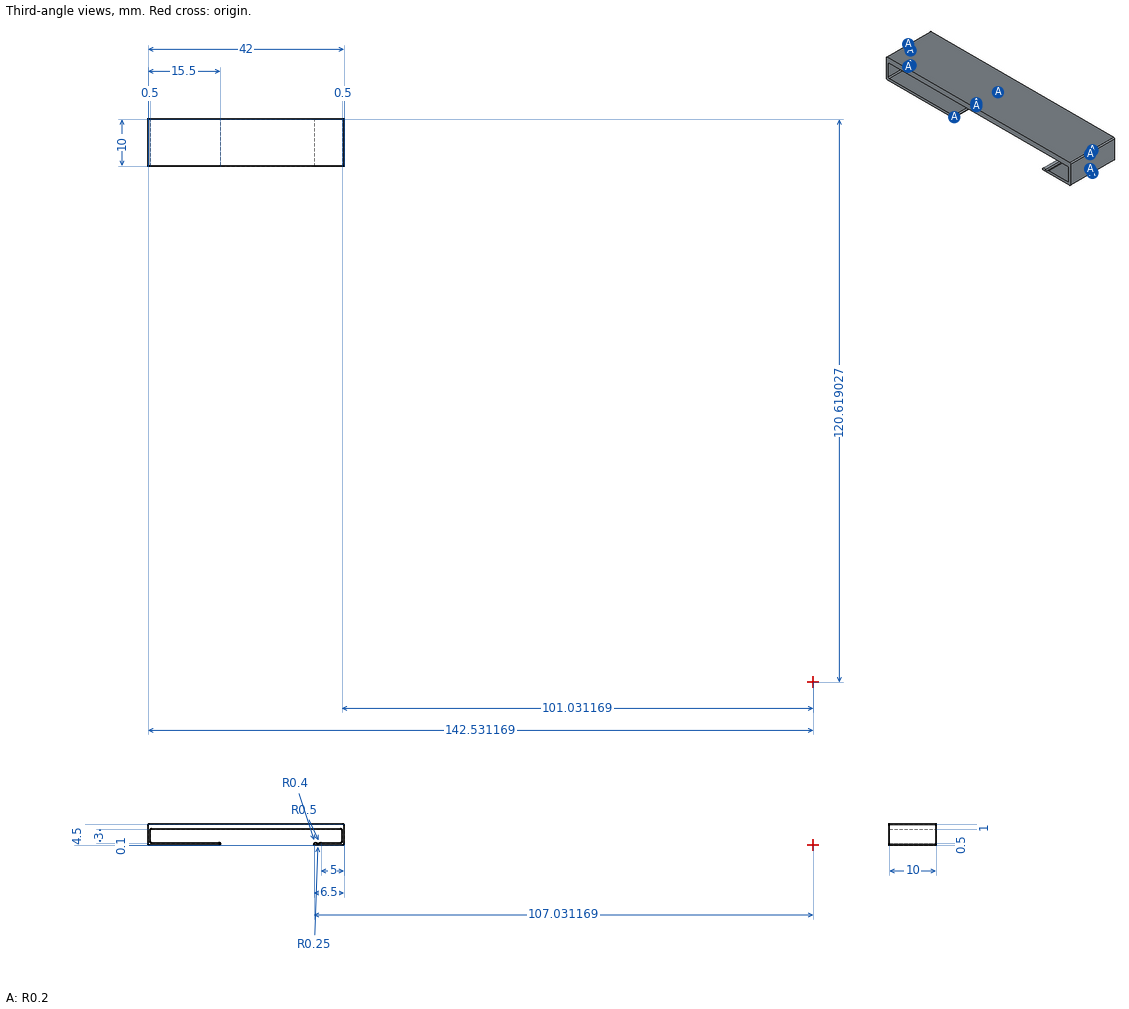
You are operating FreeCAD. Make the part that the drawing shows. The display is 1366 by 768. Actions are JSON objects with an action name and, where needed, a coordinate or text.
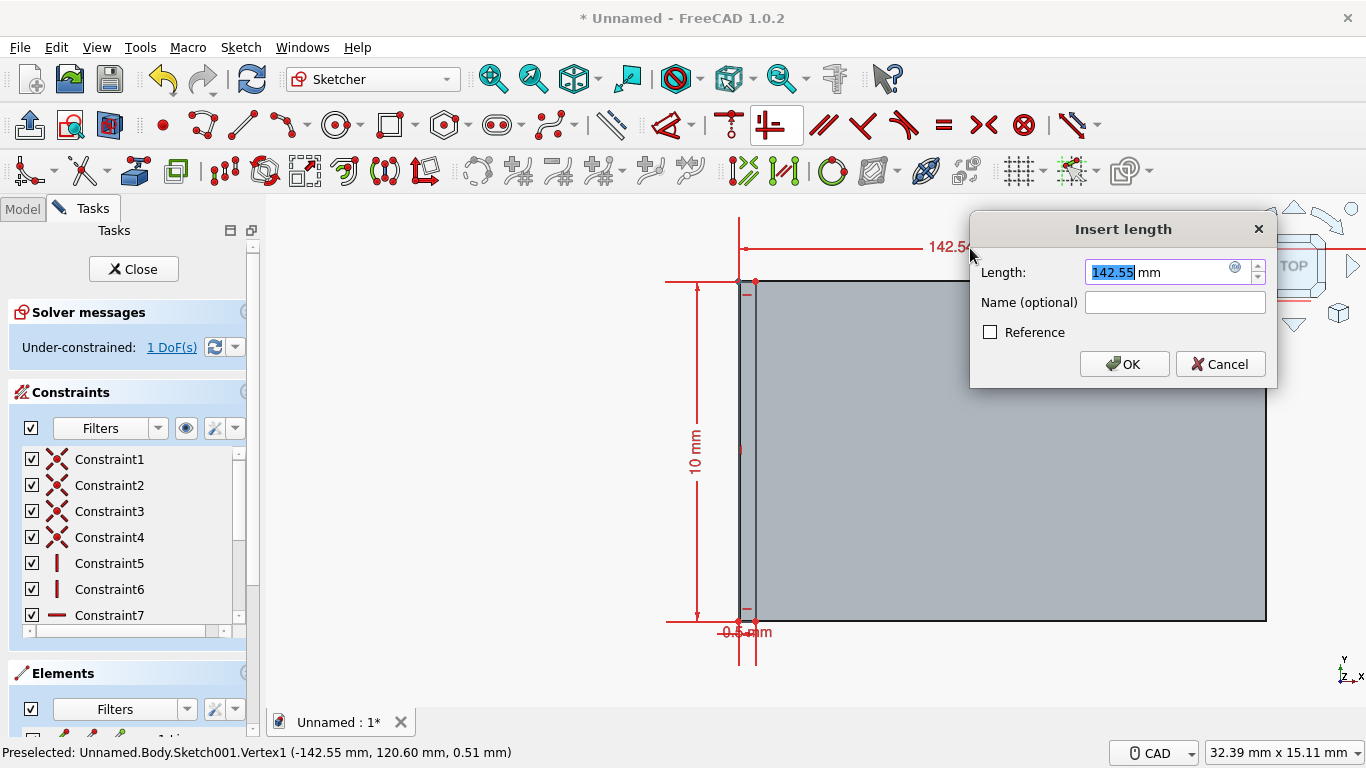
{"action": "type", "text": "142.531169"}
{"action": "key", "text": "Return"}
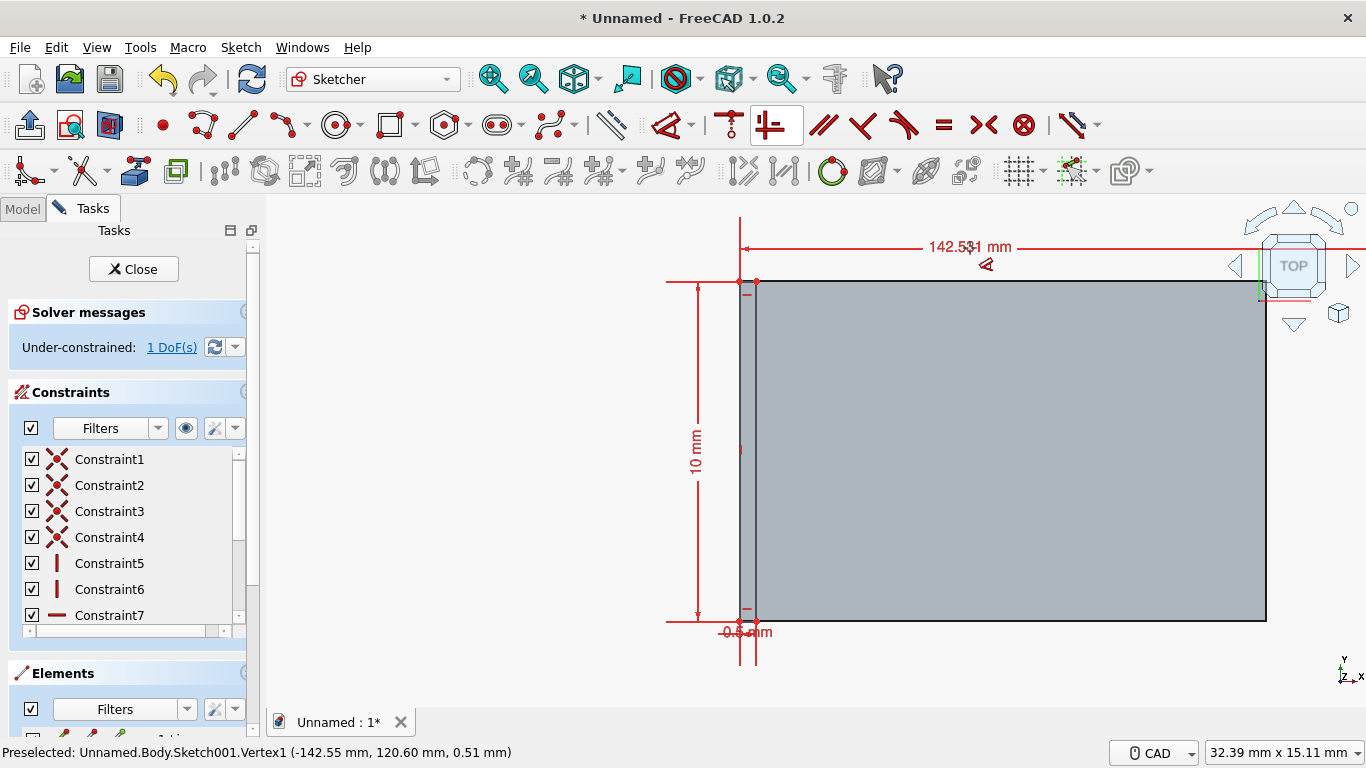
{"action": "left_click", "coordinate": [740, 282]}
{"action": "left_click", "coordinate": [706, 480]}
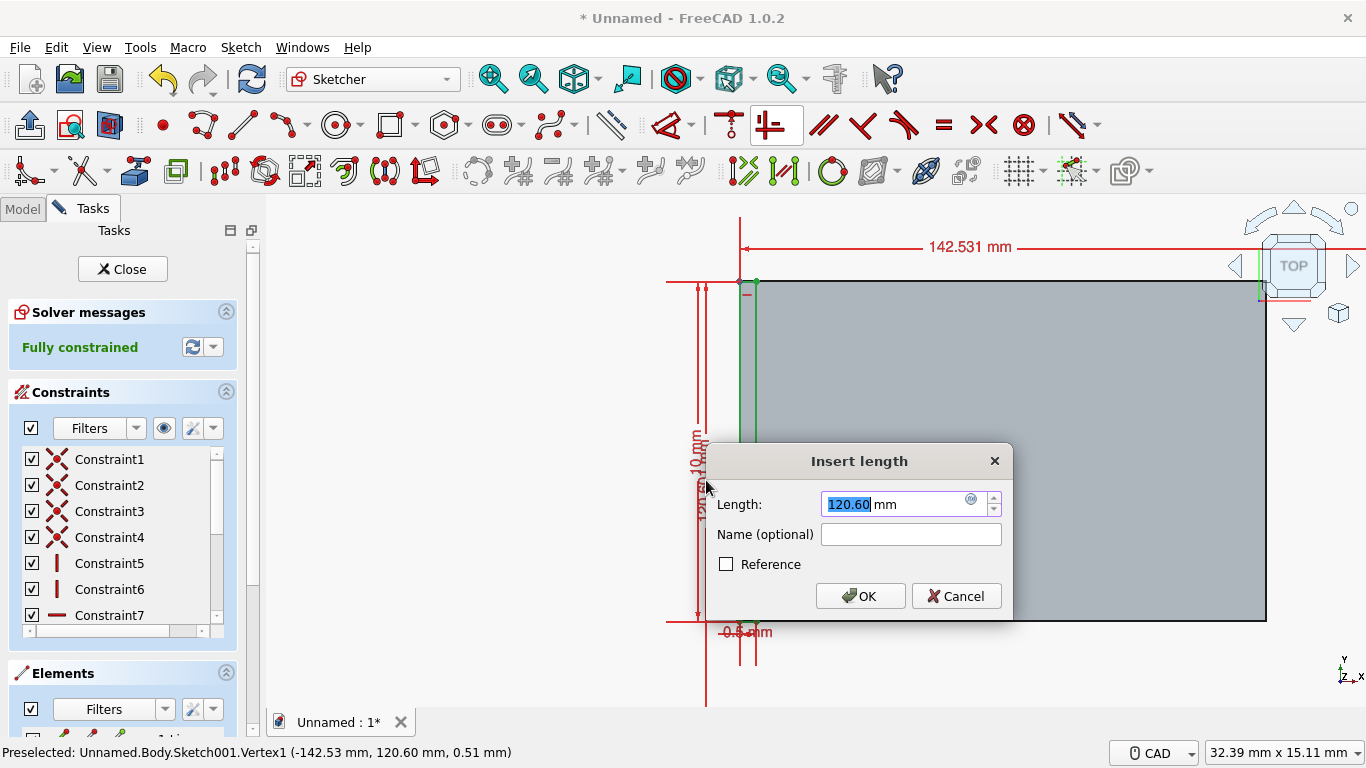
{"action": "type", "text": "120.619027"}
{"action": "key", "text": "Return"}
{"action": "key", "text": "Escape"}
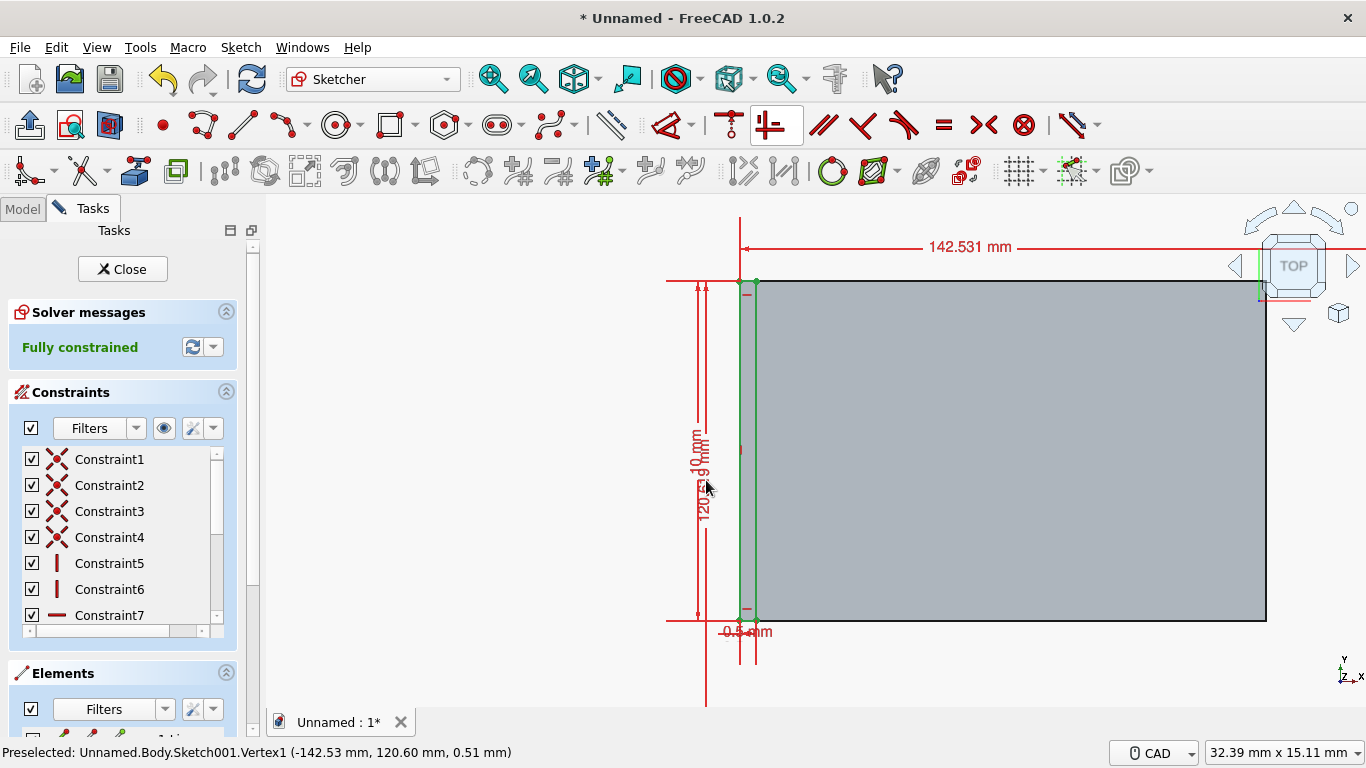
{"action": "left_click", "coordinate": [123, 269]}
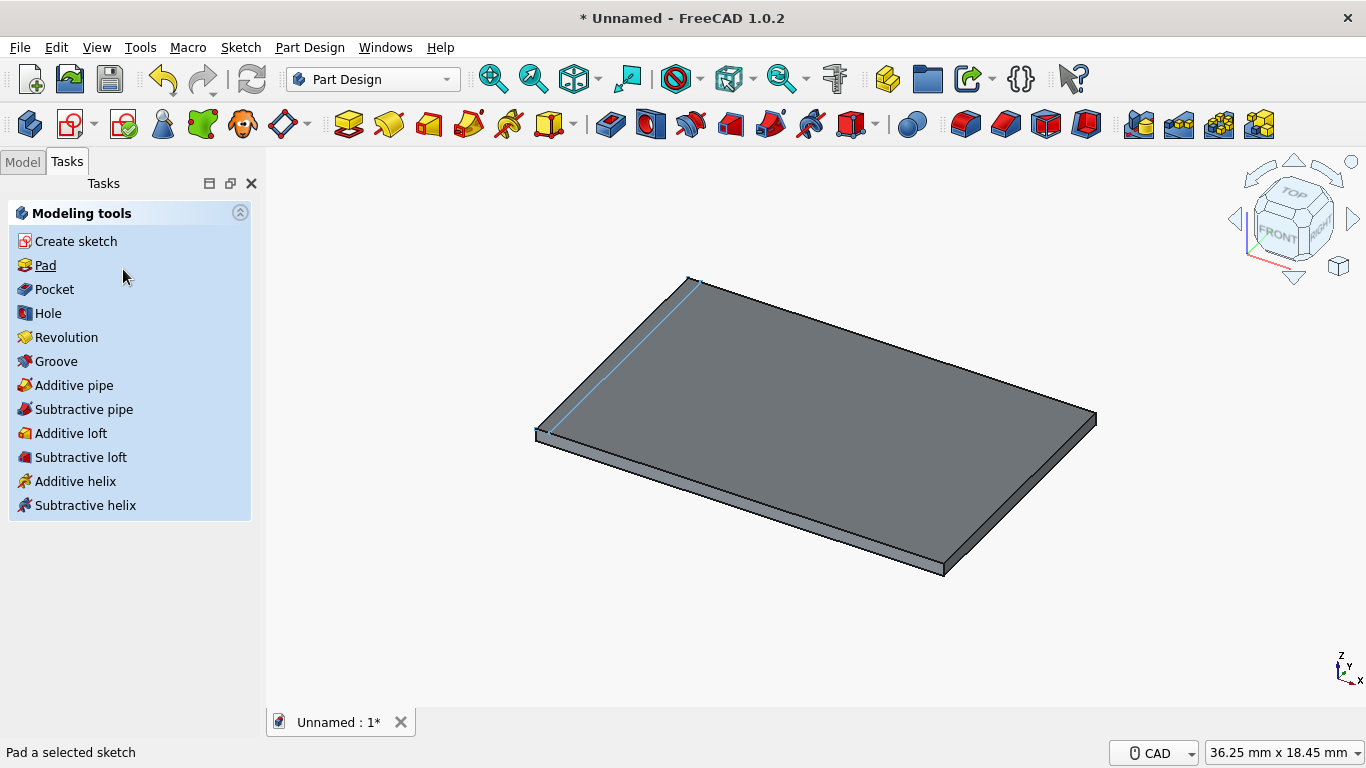
{"action": "left_click", "coordinate": [350, 124]}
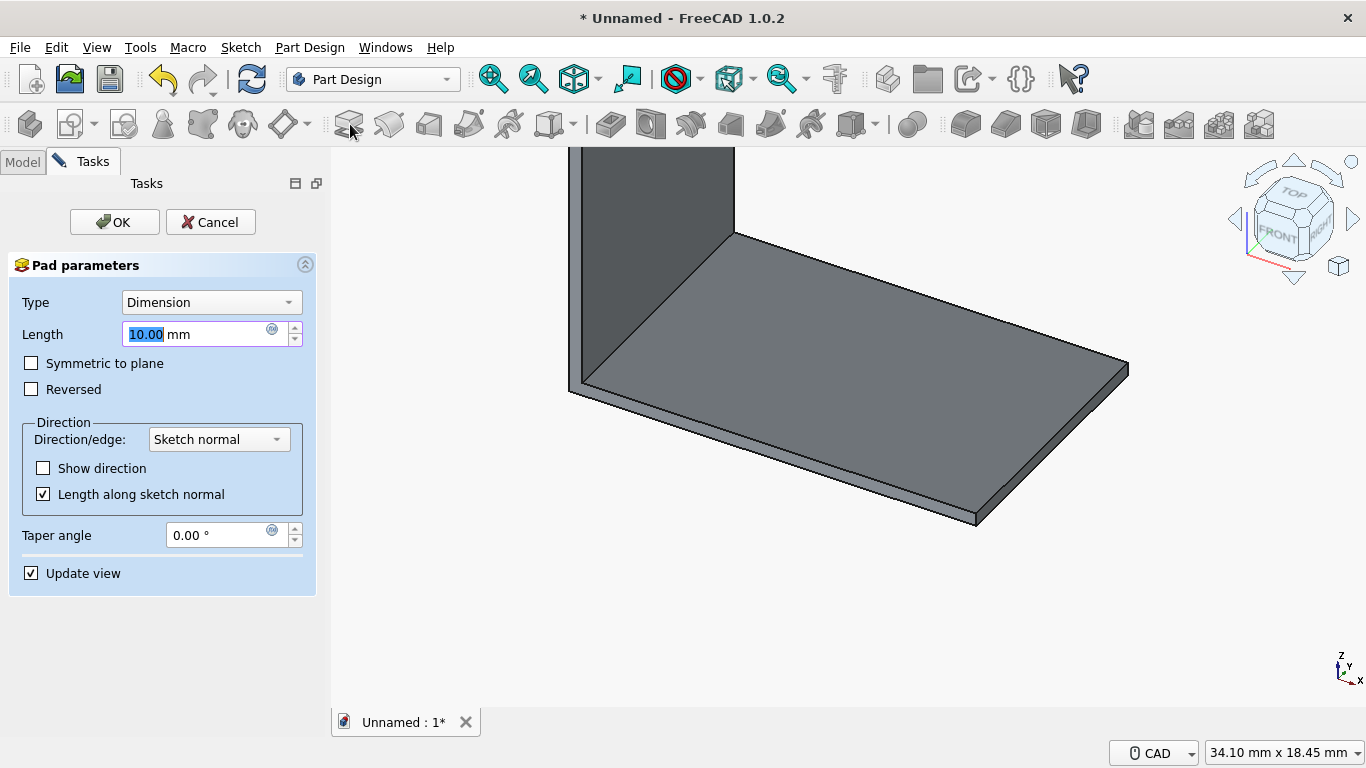
{"action": "type", "text": "3"}
{"action": "key", "text": "Tab"}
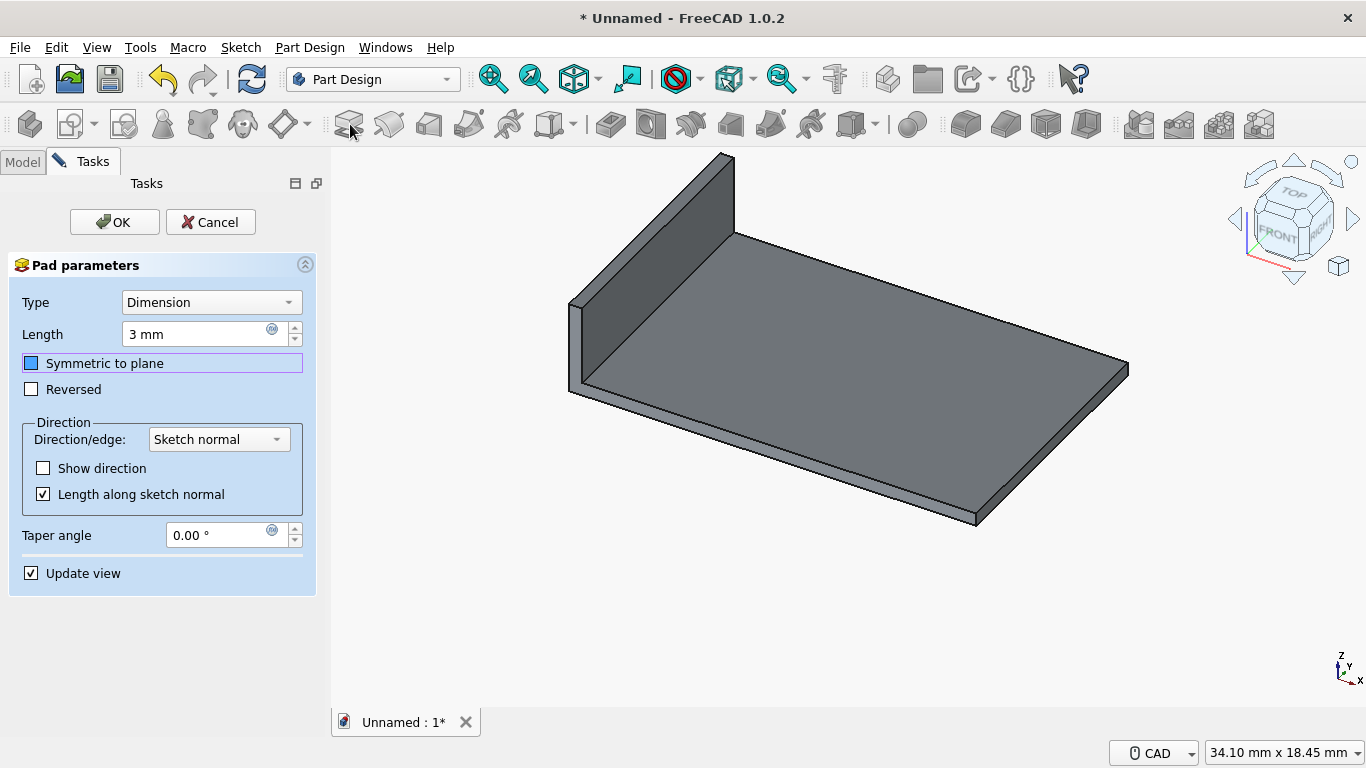
{"action": "left_click", "coordinate": [115, 222]}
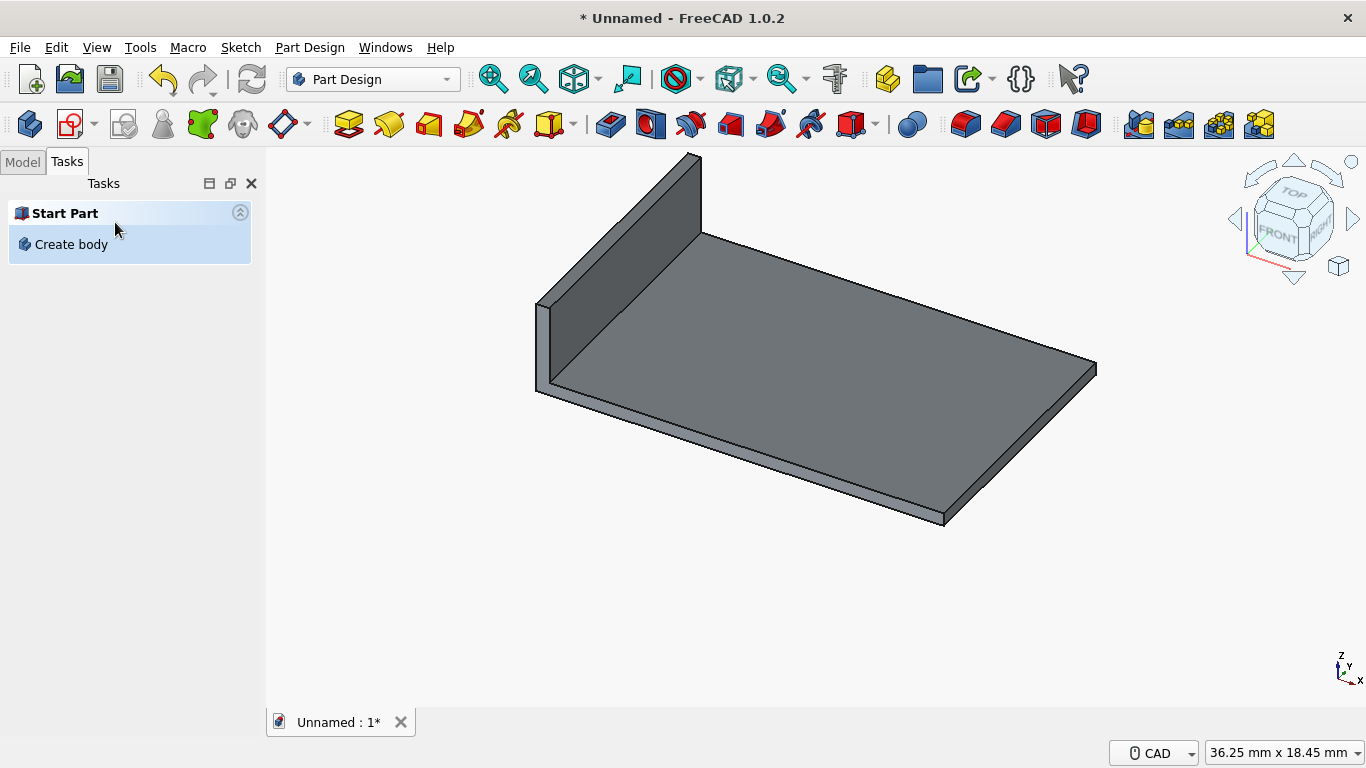
{"action": "key", "text": "0"}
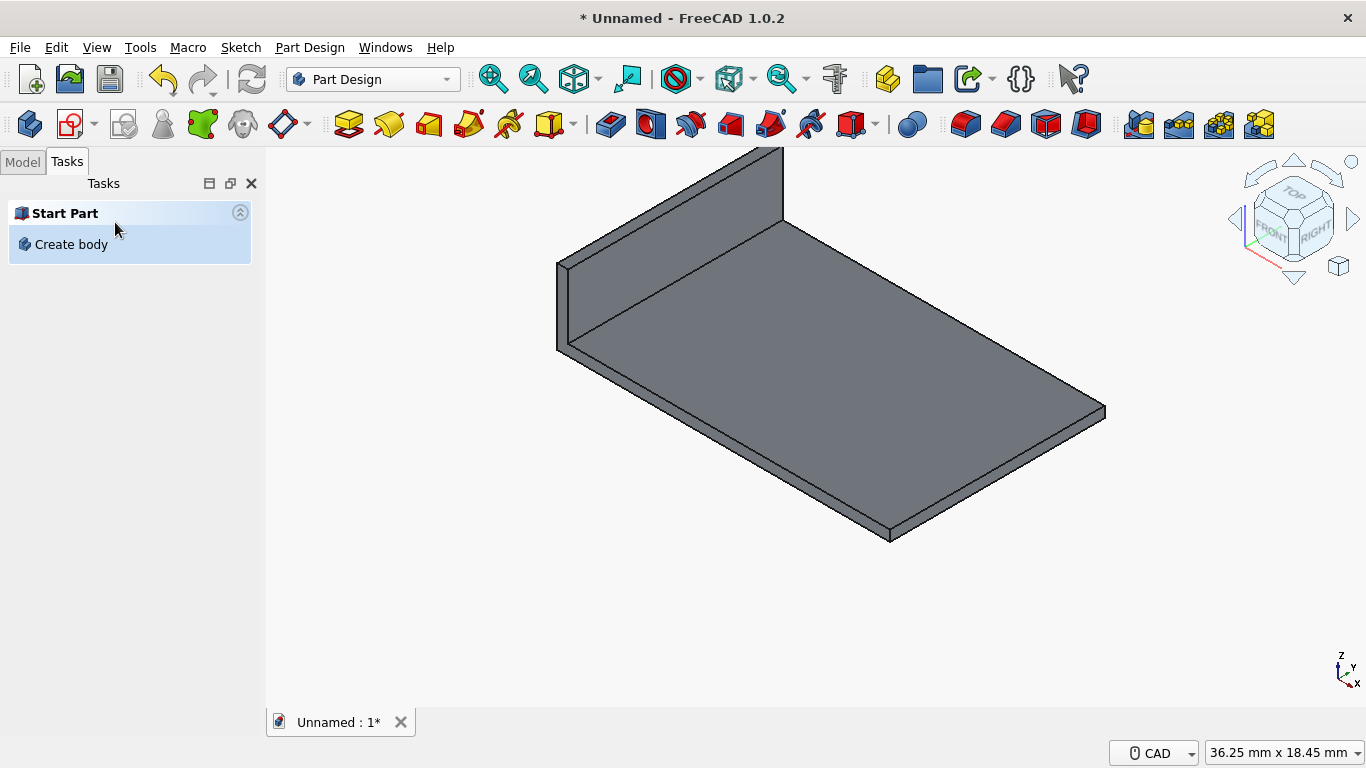
{"action": "left_click", "coordinate": [494, 80]}